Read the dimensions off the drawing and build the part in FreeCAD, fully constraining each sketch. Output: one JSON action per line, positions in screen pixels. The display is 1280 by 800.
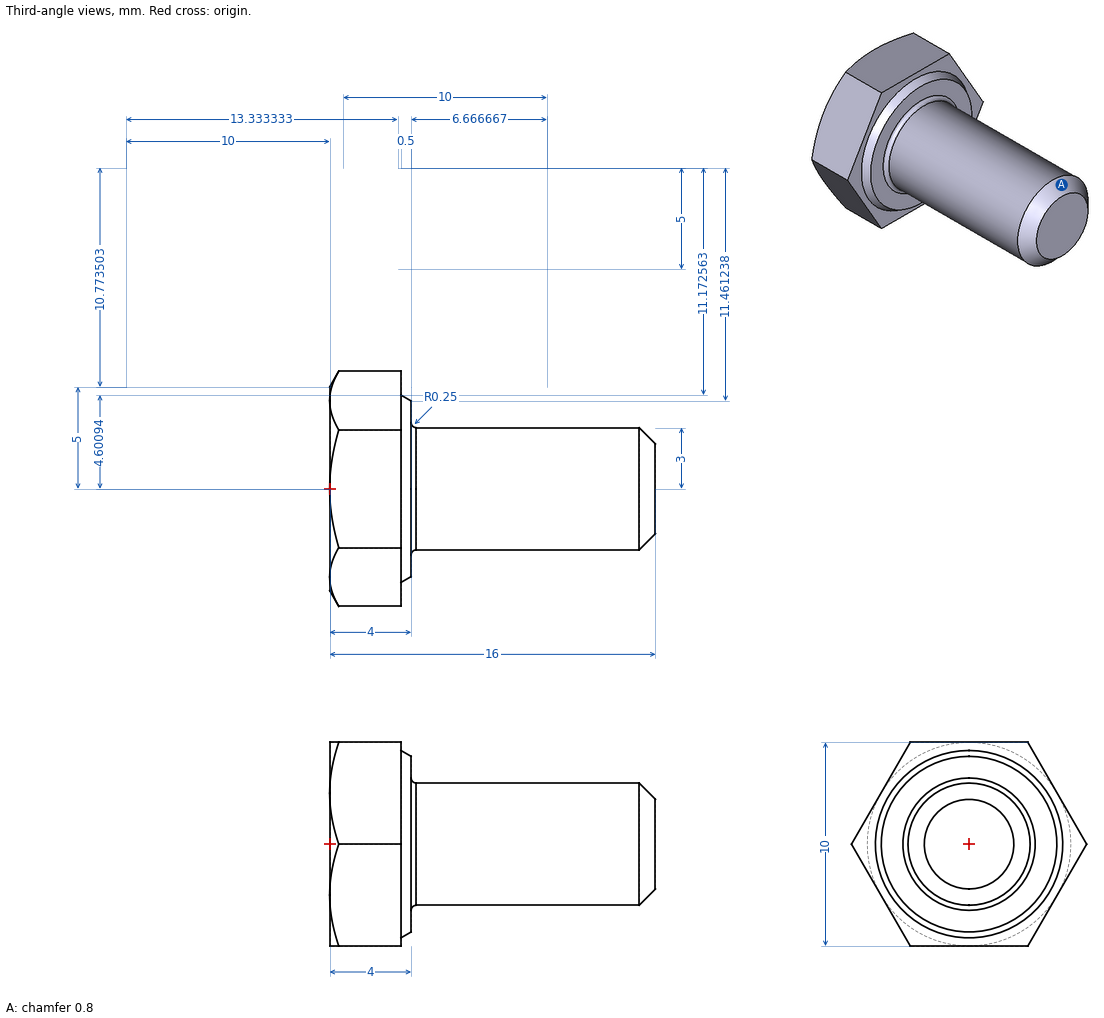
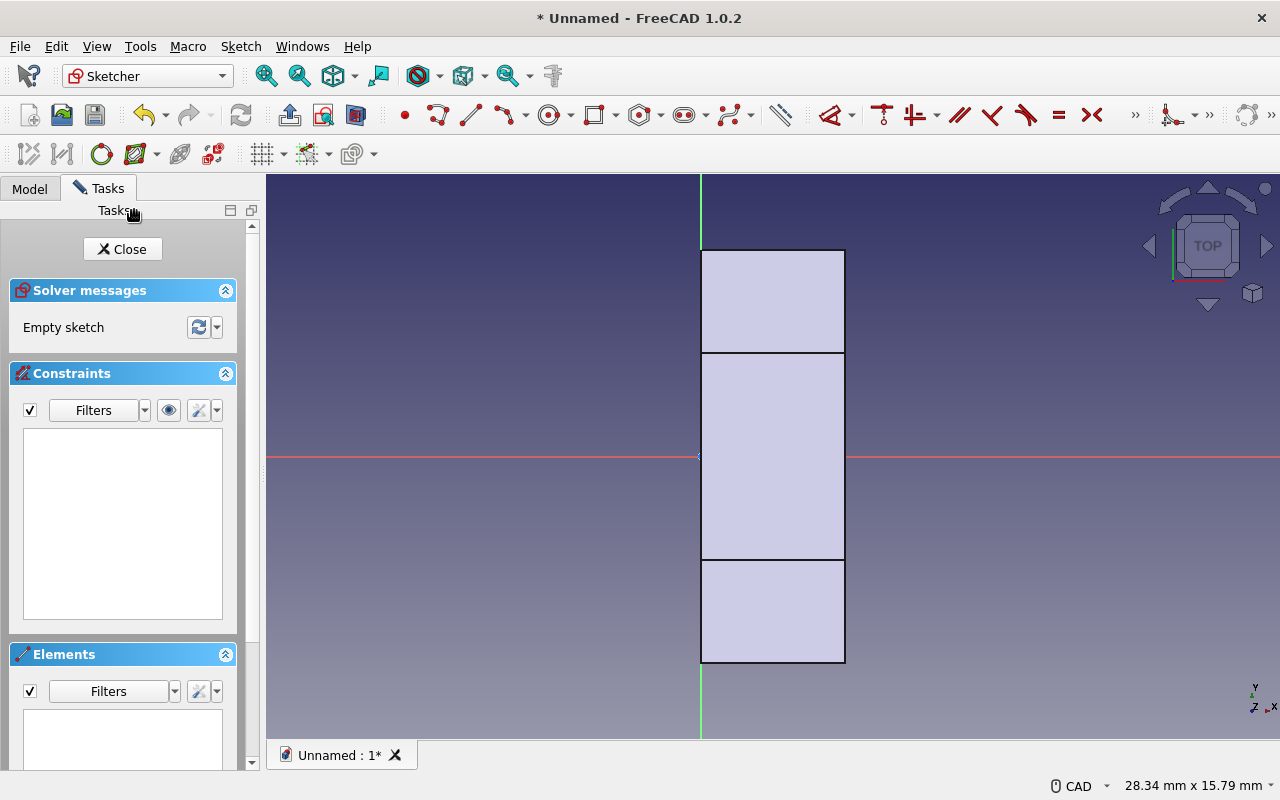
{"action": "left_click", "coordinate": [356, 116]}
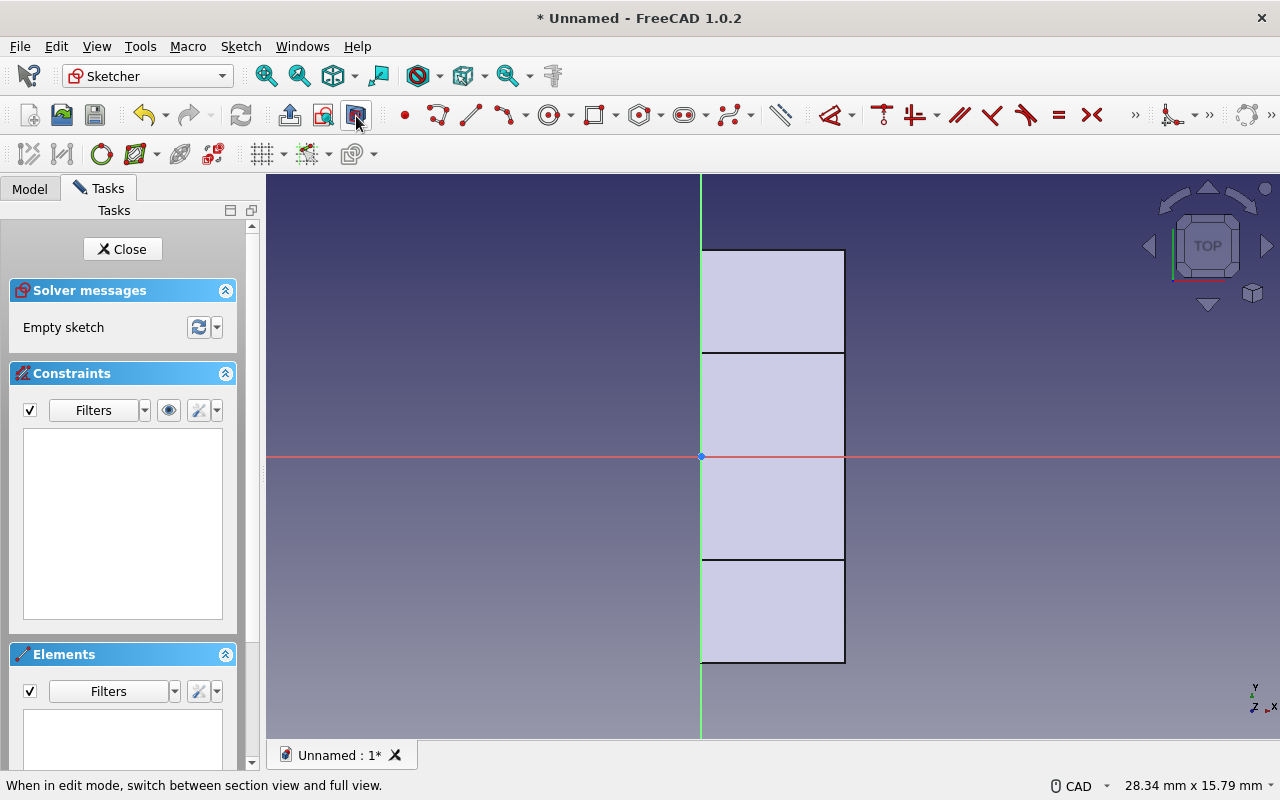
{"action": "scroll", "coordinate": [294, 566], "scroll_direction": "down", "scroll_amount": 2}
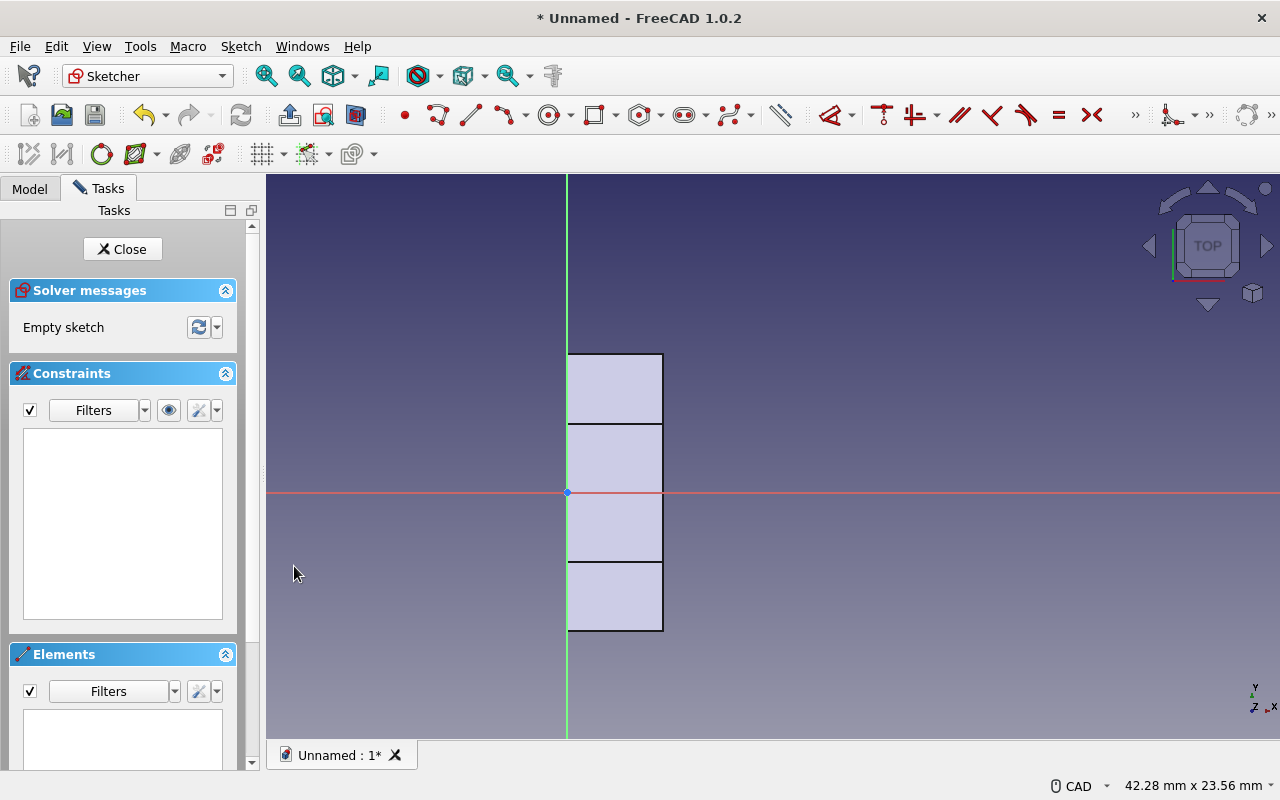
{"action": "scroll", "coordinate": [870, 458], "scroll_direction": "up", "scroll_amount": 2}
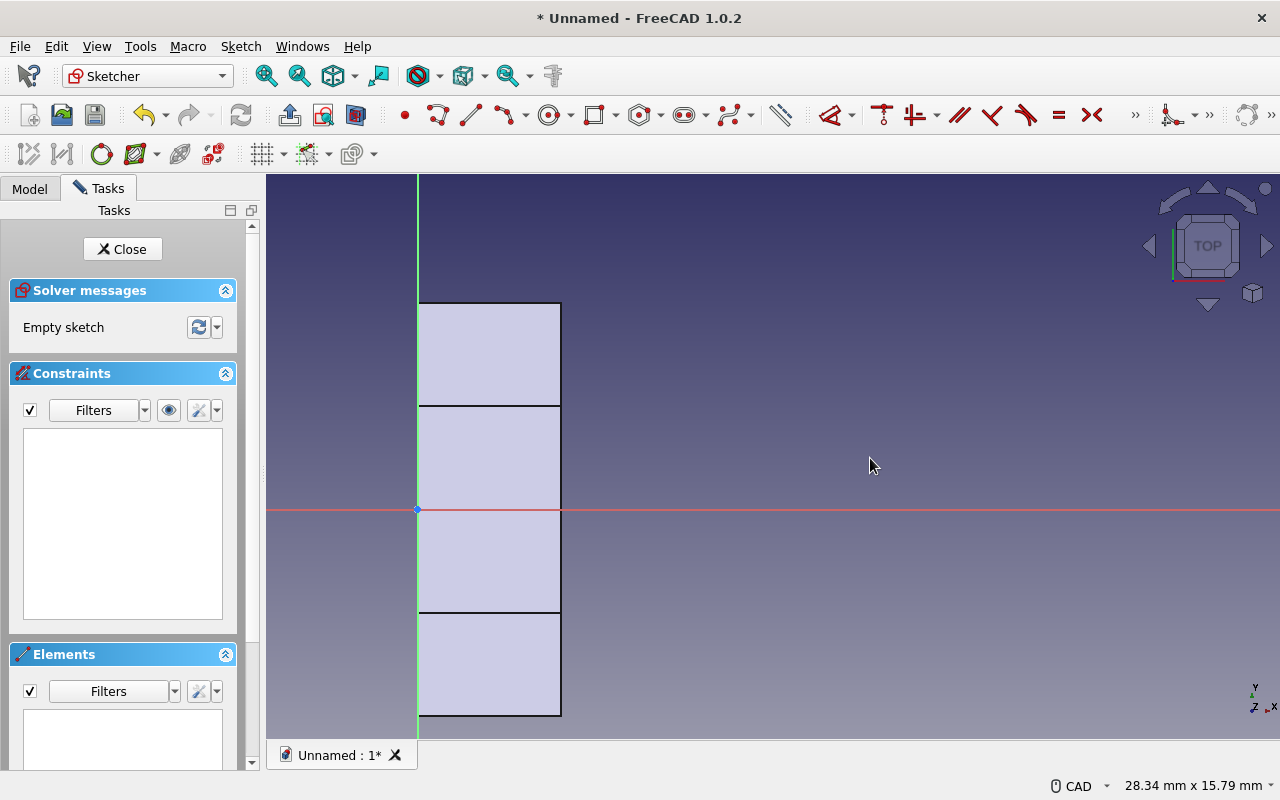
{"action": "left_click", "coordinate": [594, 116]}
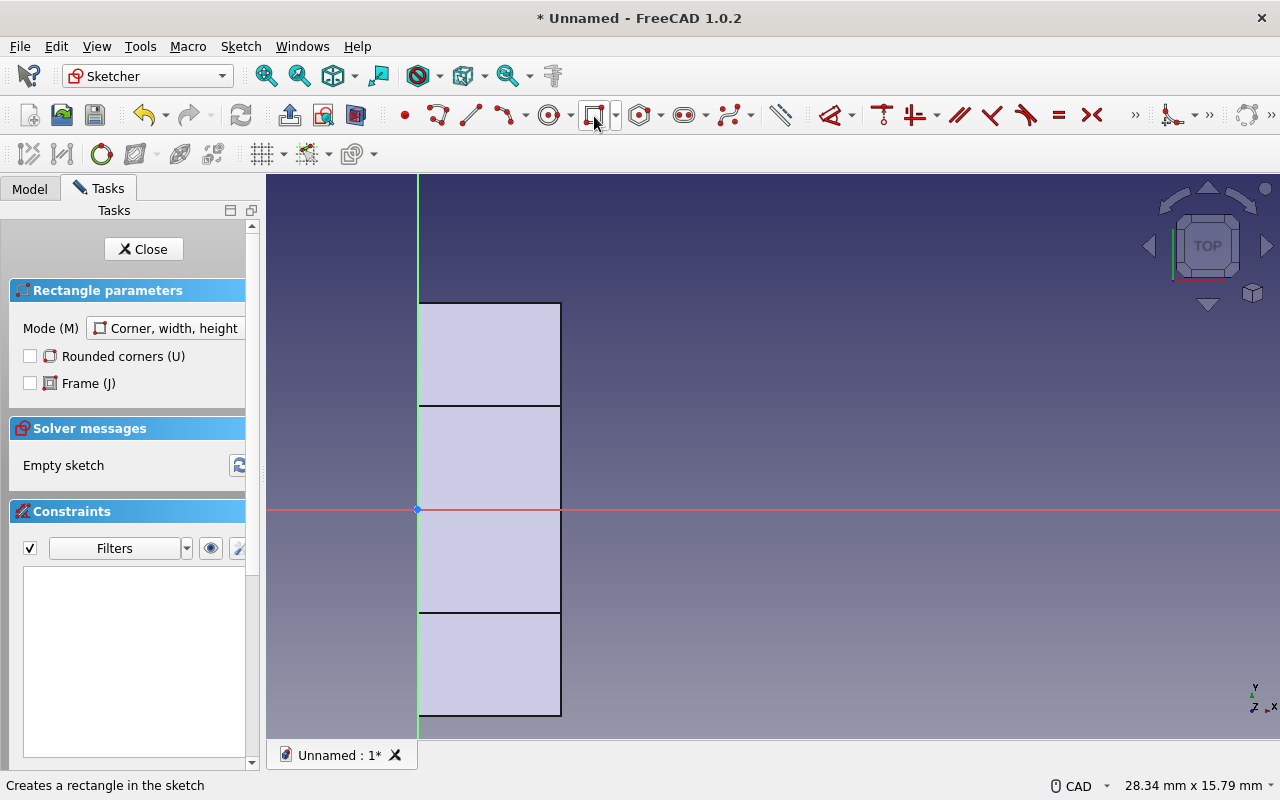
{"action": "left_click", "coordinate": [418, 510]}
{"action": "mouse_move", "coordinate": [990, 402]}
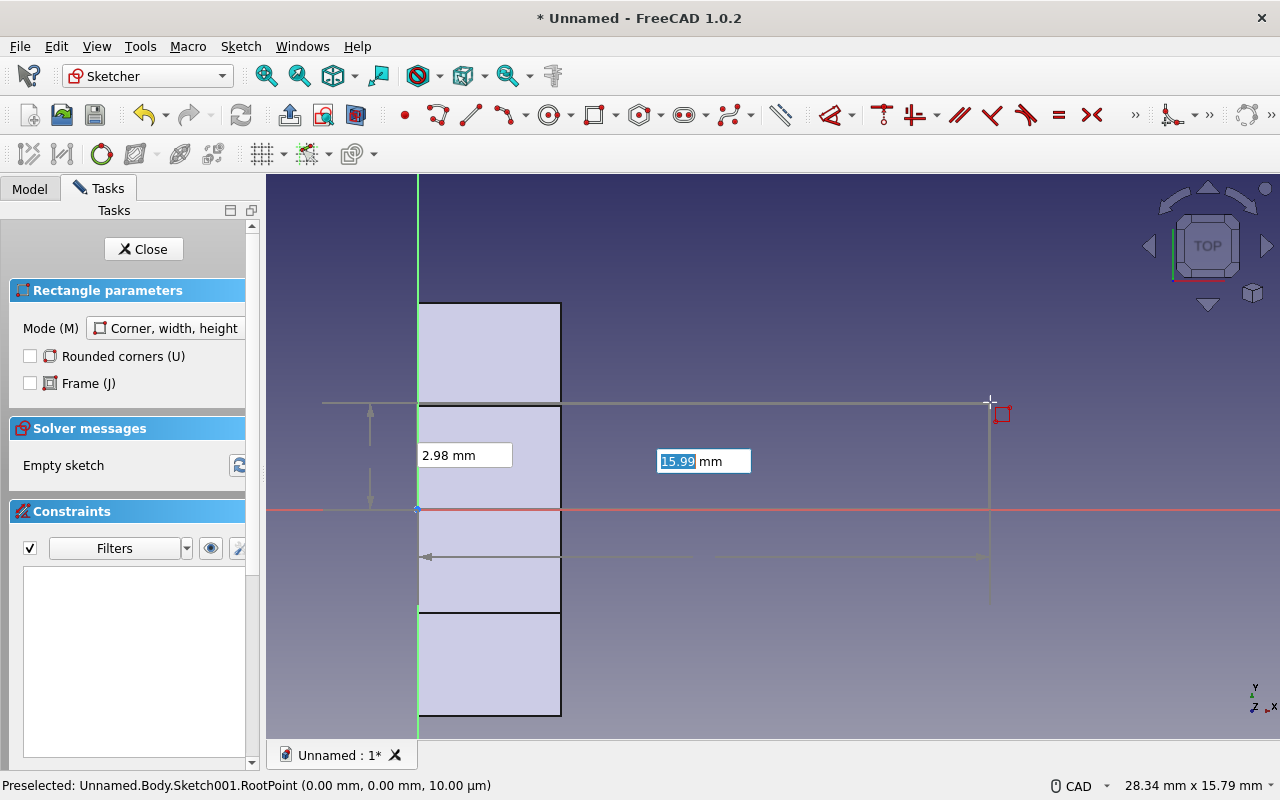
{"action": "type", "text": "16"}
{"action": "key", "text": "Tab"}
{"action": "type", "text": "3"}
{"action": "key", "text": "Return"}
{"action": "key", "text": "Escape"}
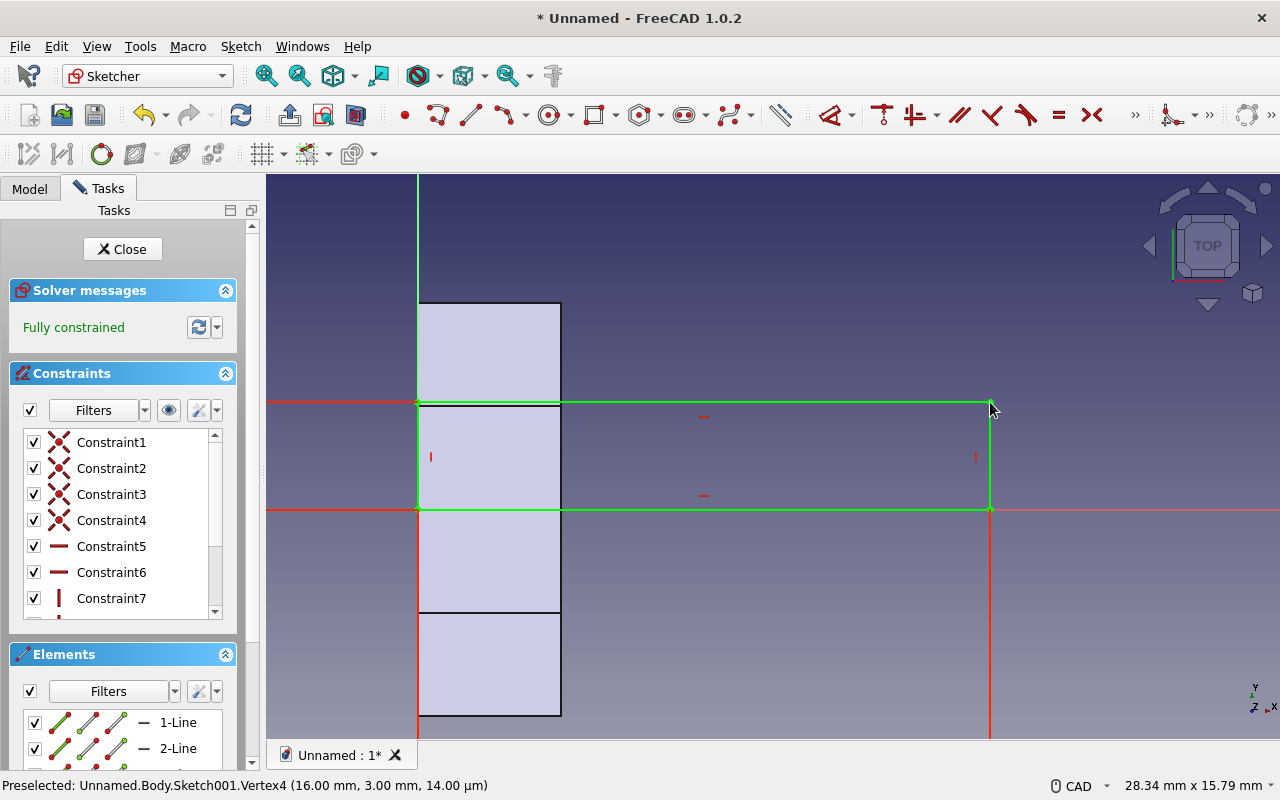
{"action": "left_click", "coordinate": [123, 249]}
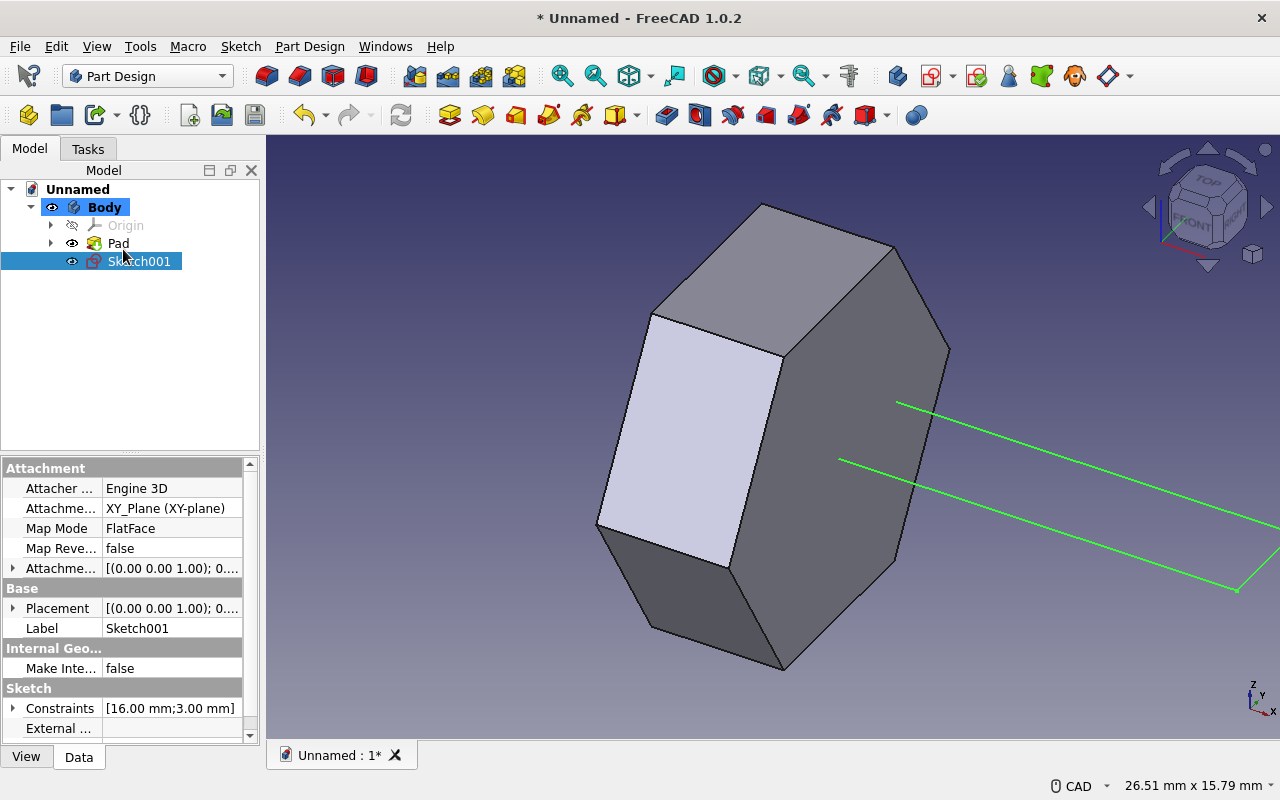
{"action": "left_click", "coordinate": [483, 116]}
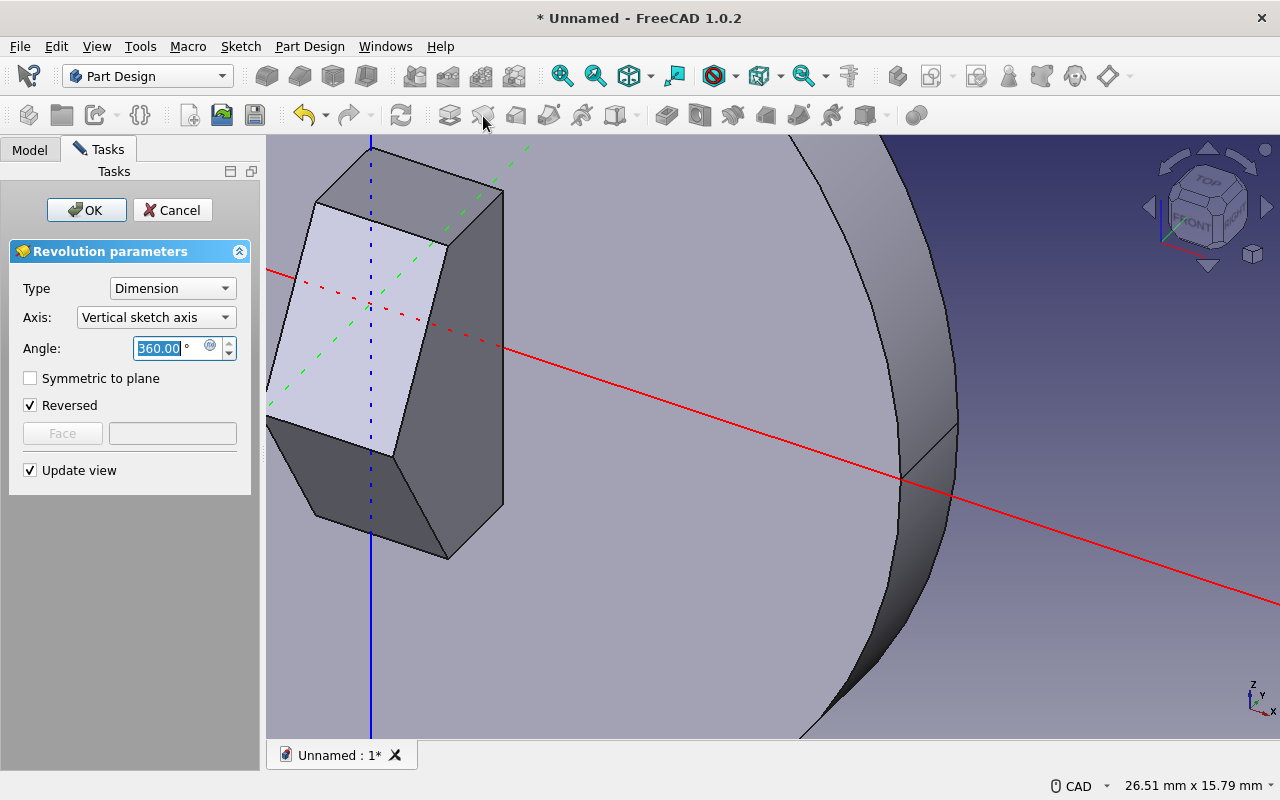
{"action": "left_click", "coordinate": [157, 318]}